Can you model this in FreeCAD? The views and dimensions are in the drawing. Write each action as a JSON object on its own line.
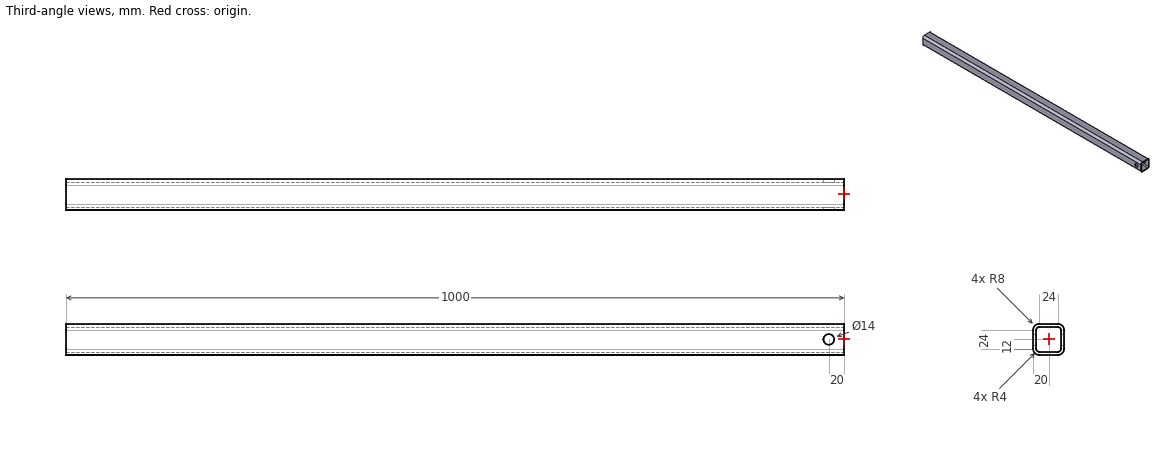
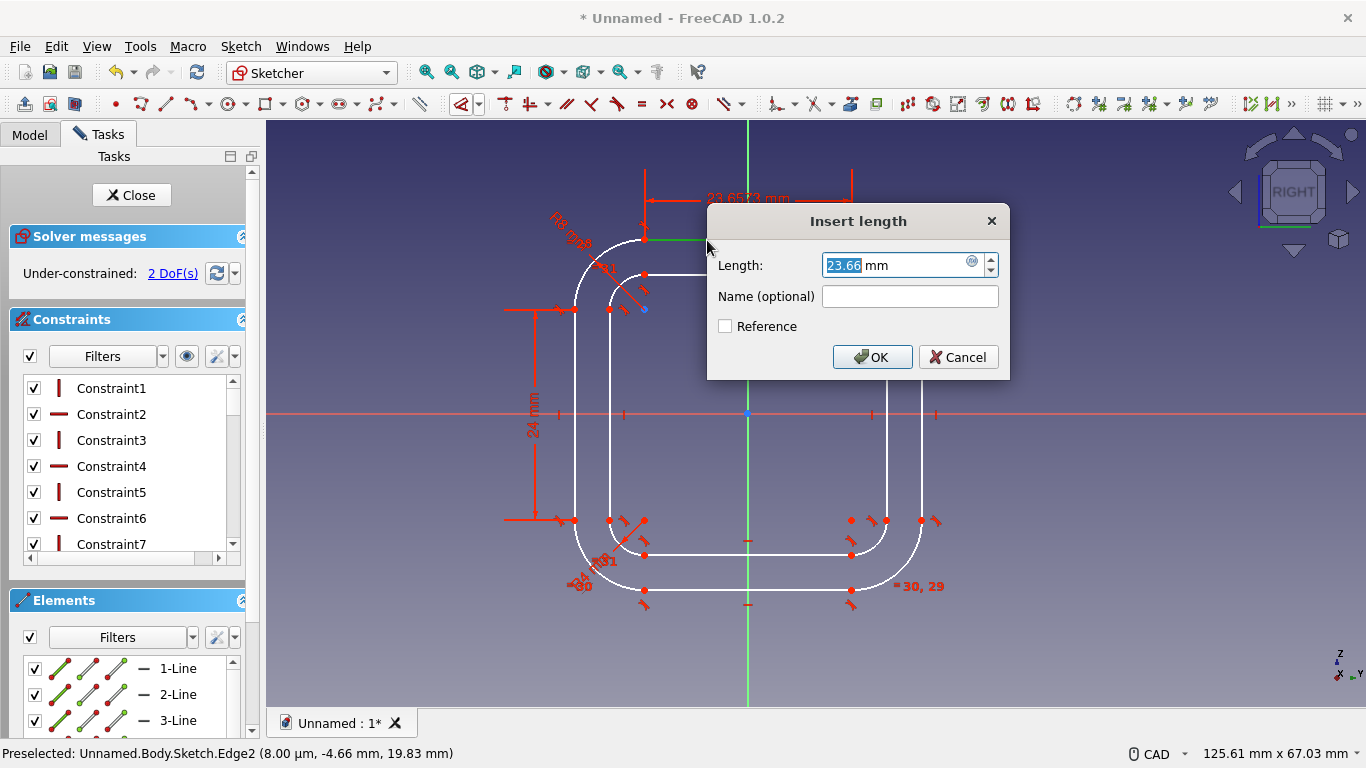
{"action": "type", "text": "24"}
{"action": "key", "text": "Return"}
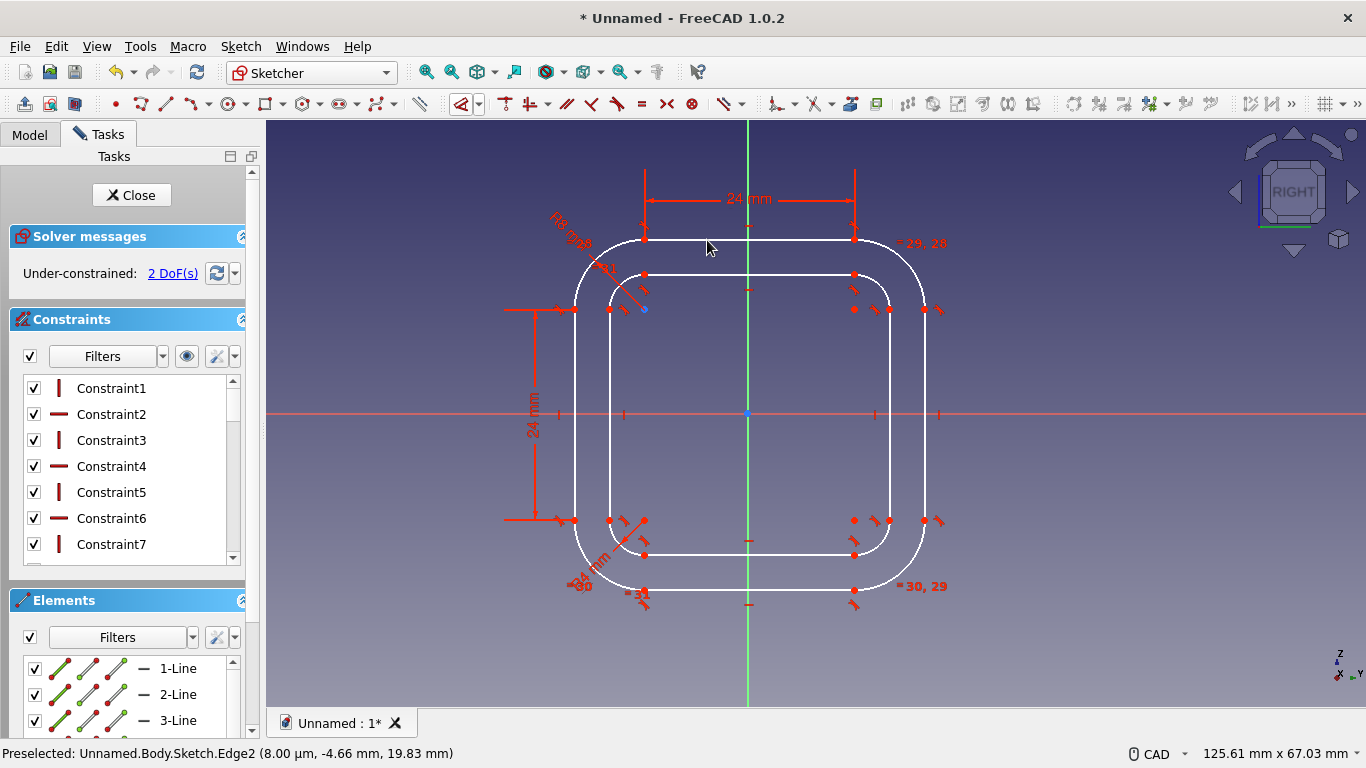
{"action": "left_click", "coordinate": [575, 520]}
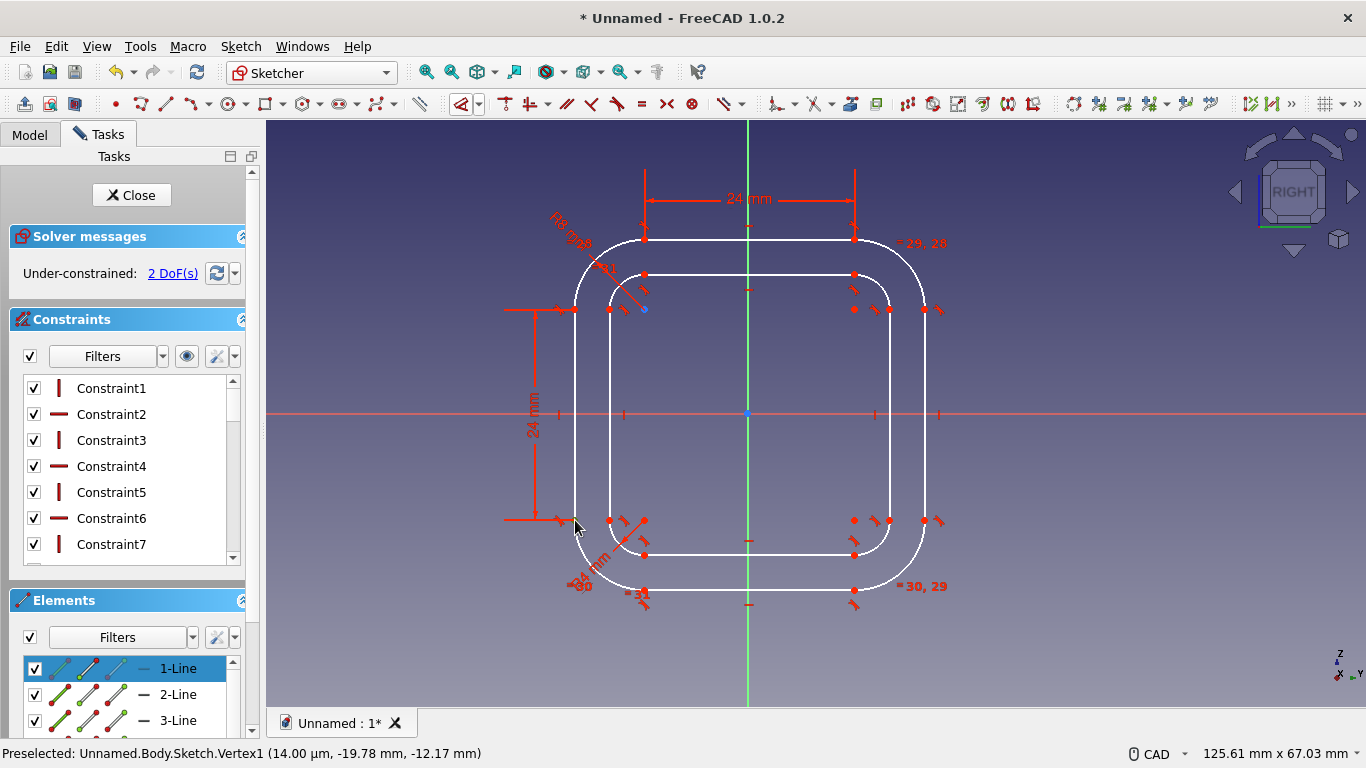
{"action": "key", "text": "l"}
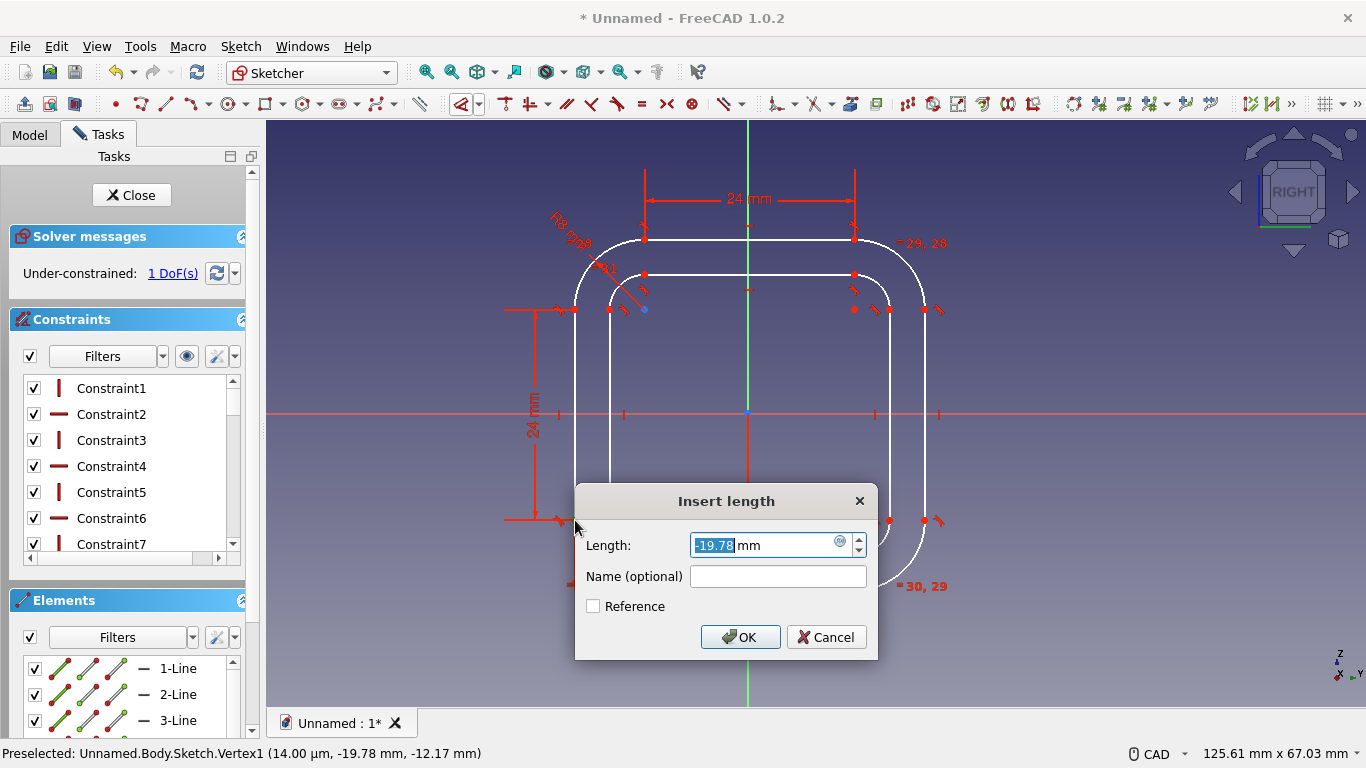
{"action": "type", "text": "-20"}
{"action": "key", "text": "Return"}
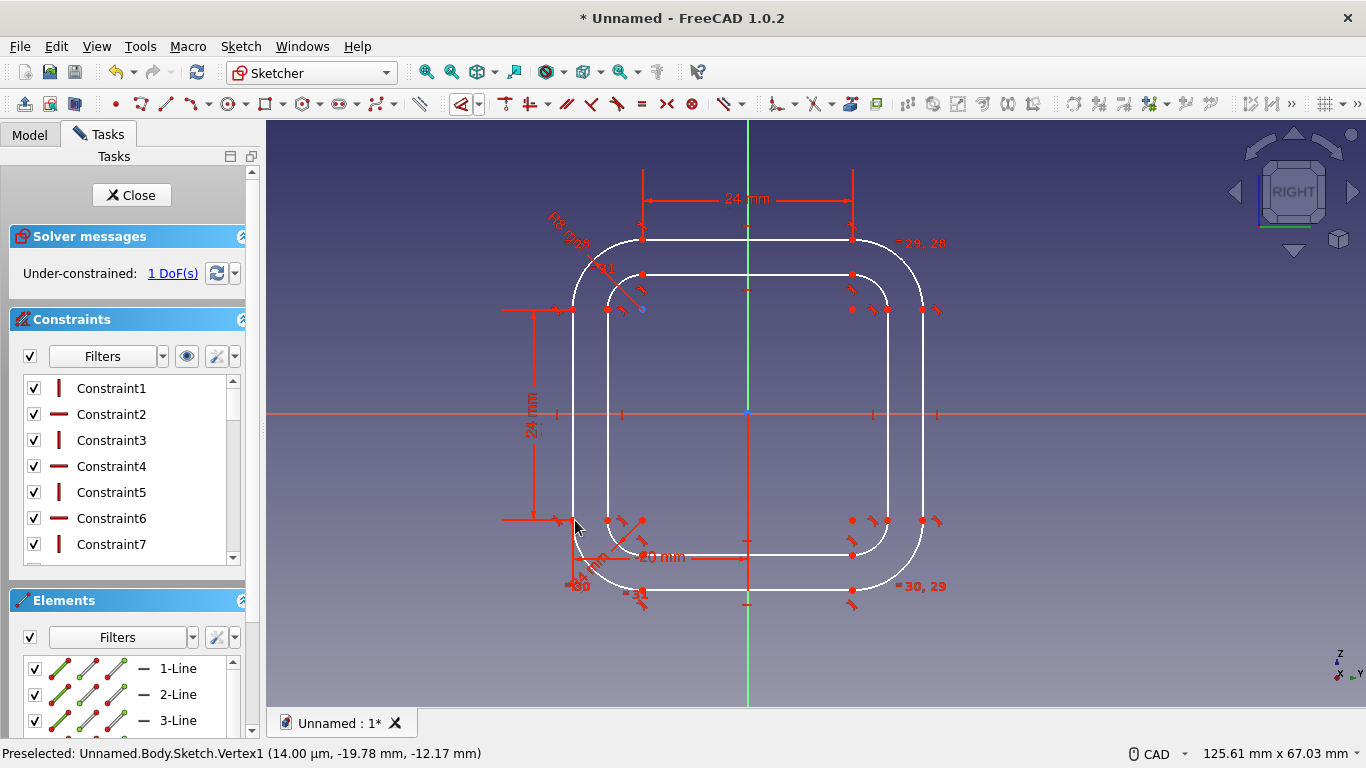
{"action": "left_click", "coordinate": [573, 520]}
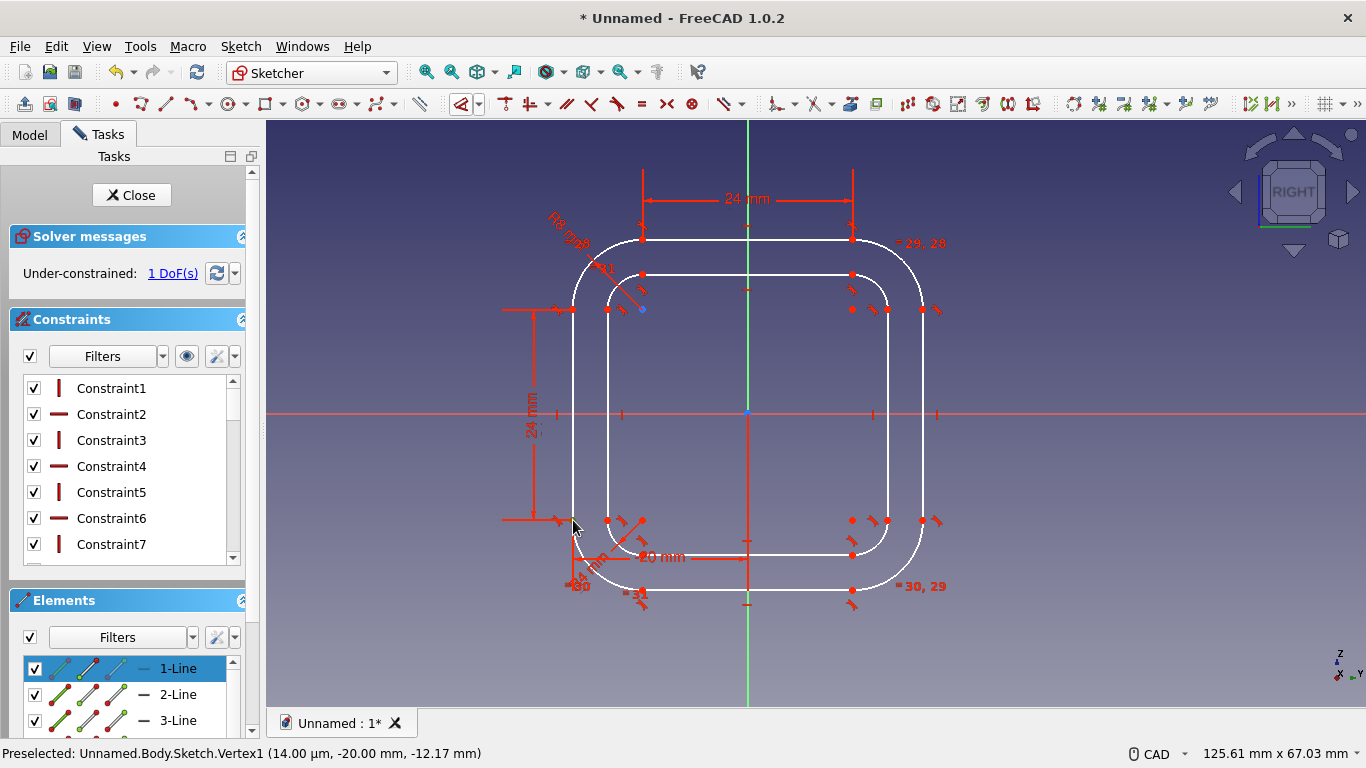
{"action": "left_click", "coordinate": [478, 104]}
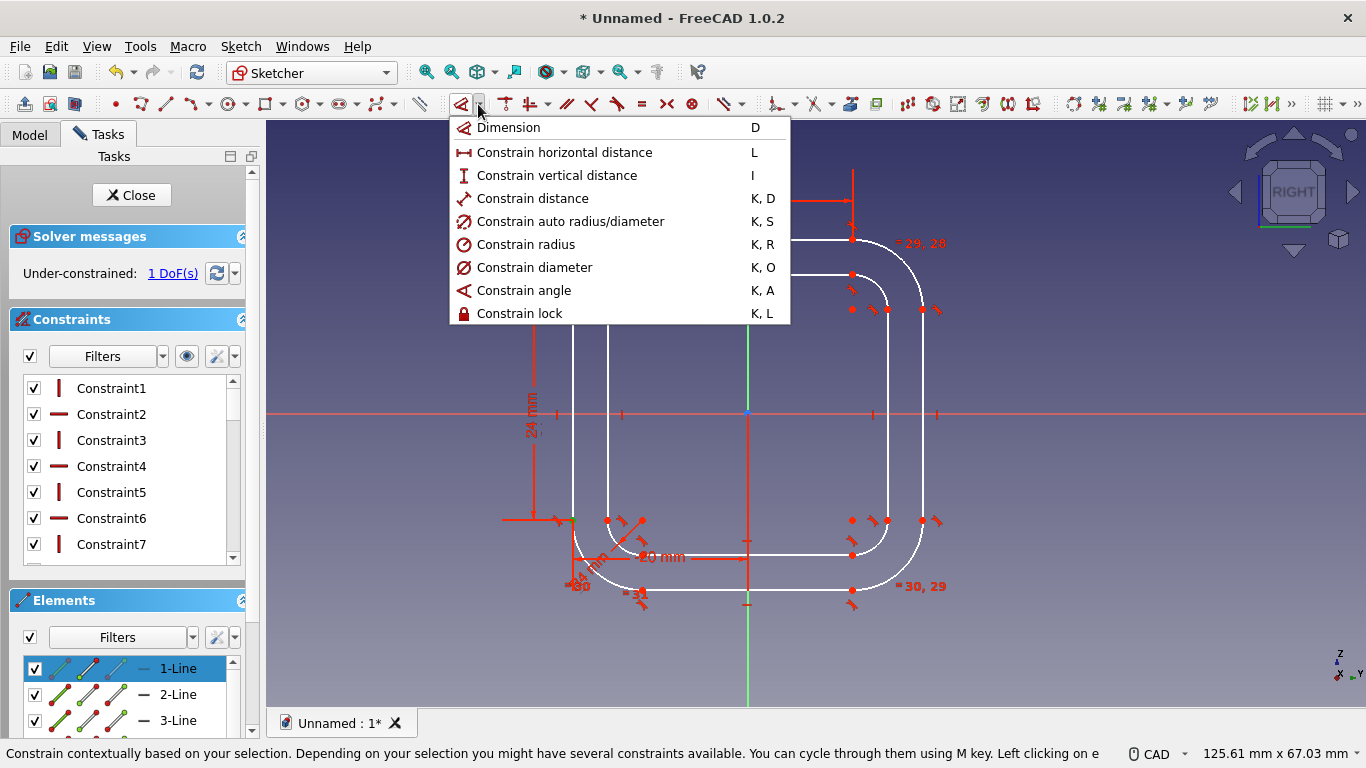
{"action": "left_click", "coordinate": [620, 176]}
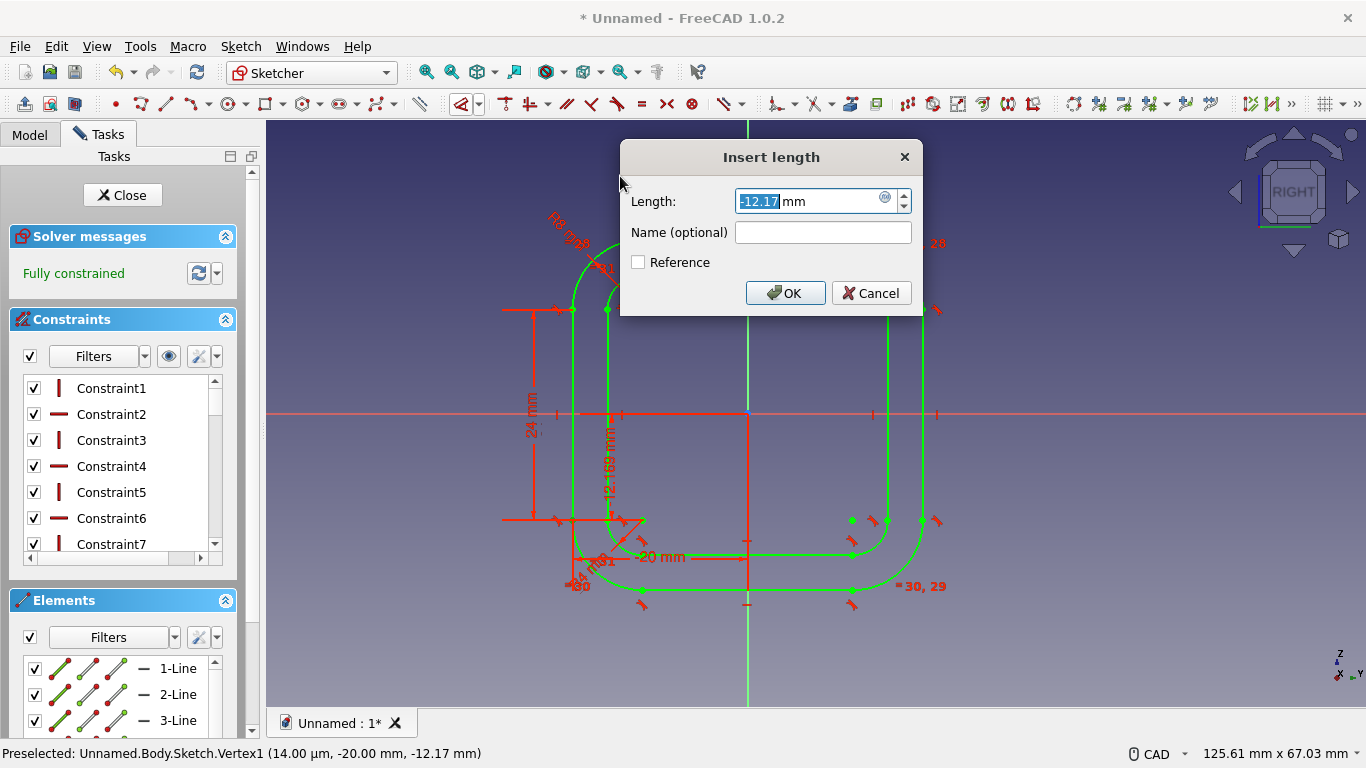
{"action": "type", "text": "-12"}
{"action": "key", "text": "Return"}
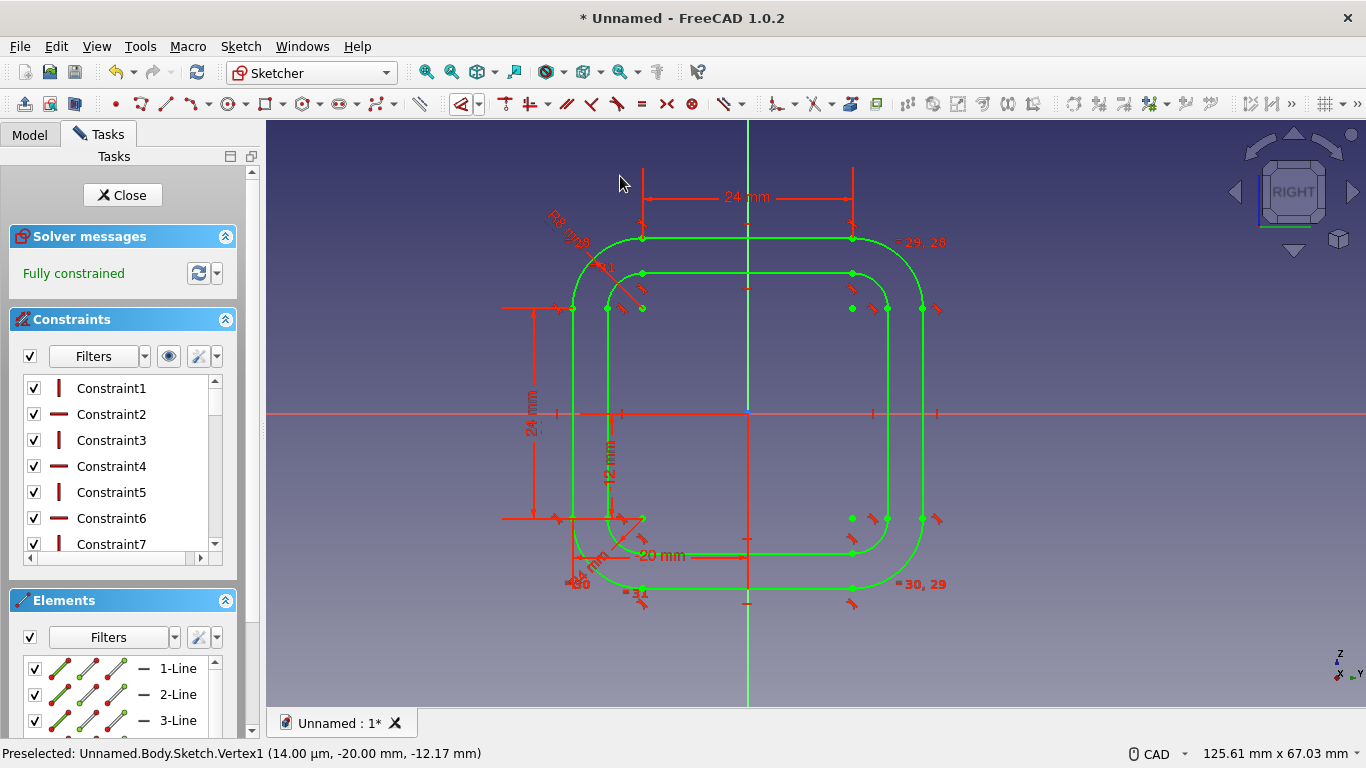
{"action": "left_click", "coordinate": [123, 195]}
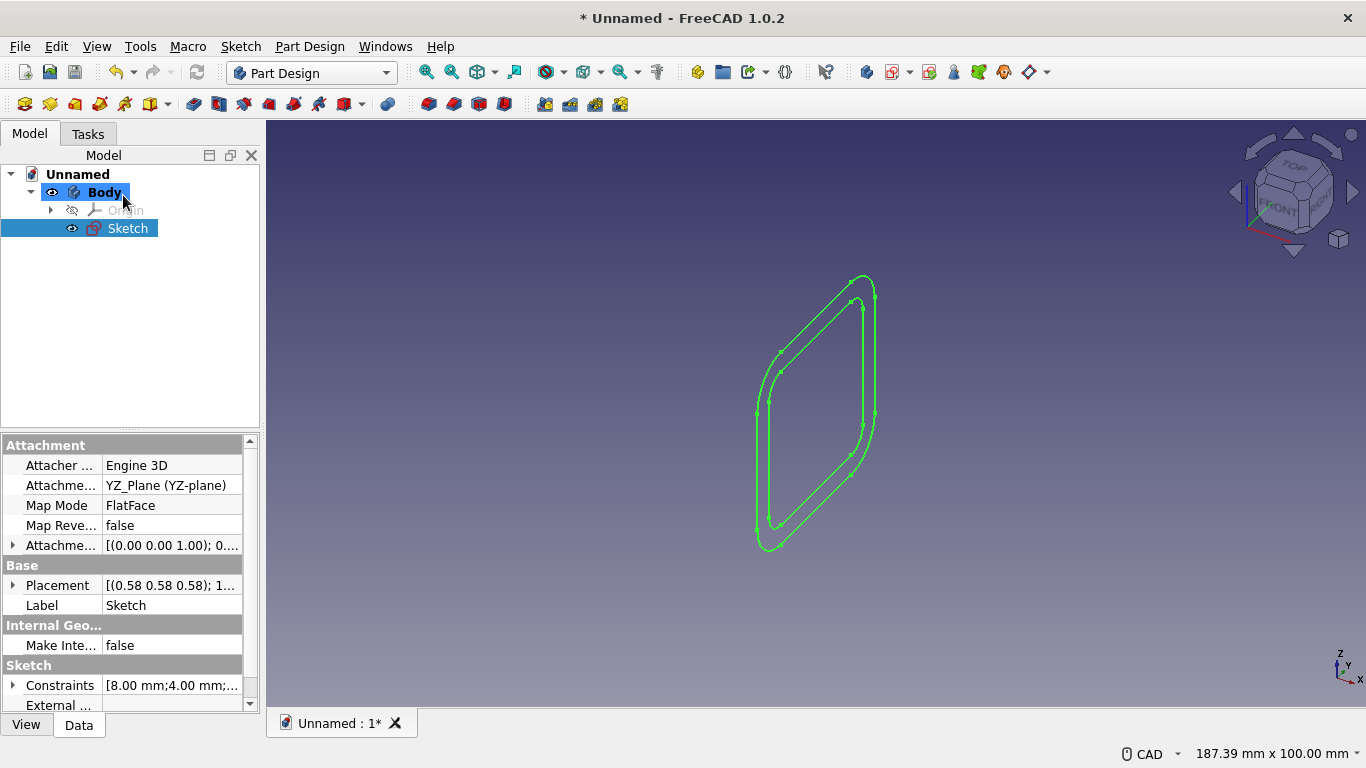
{"action": "left_click", "coordinate": [25, 104]}